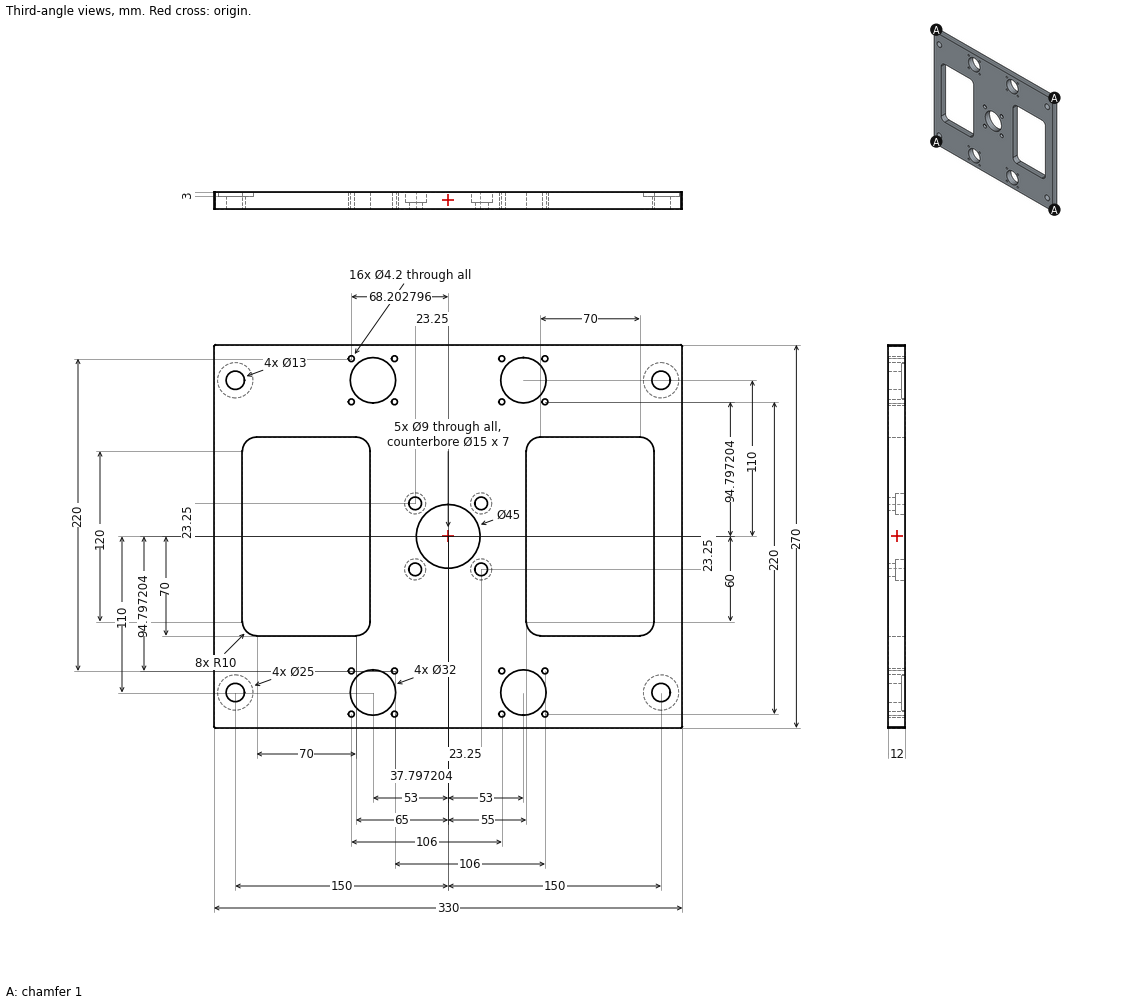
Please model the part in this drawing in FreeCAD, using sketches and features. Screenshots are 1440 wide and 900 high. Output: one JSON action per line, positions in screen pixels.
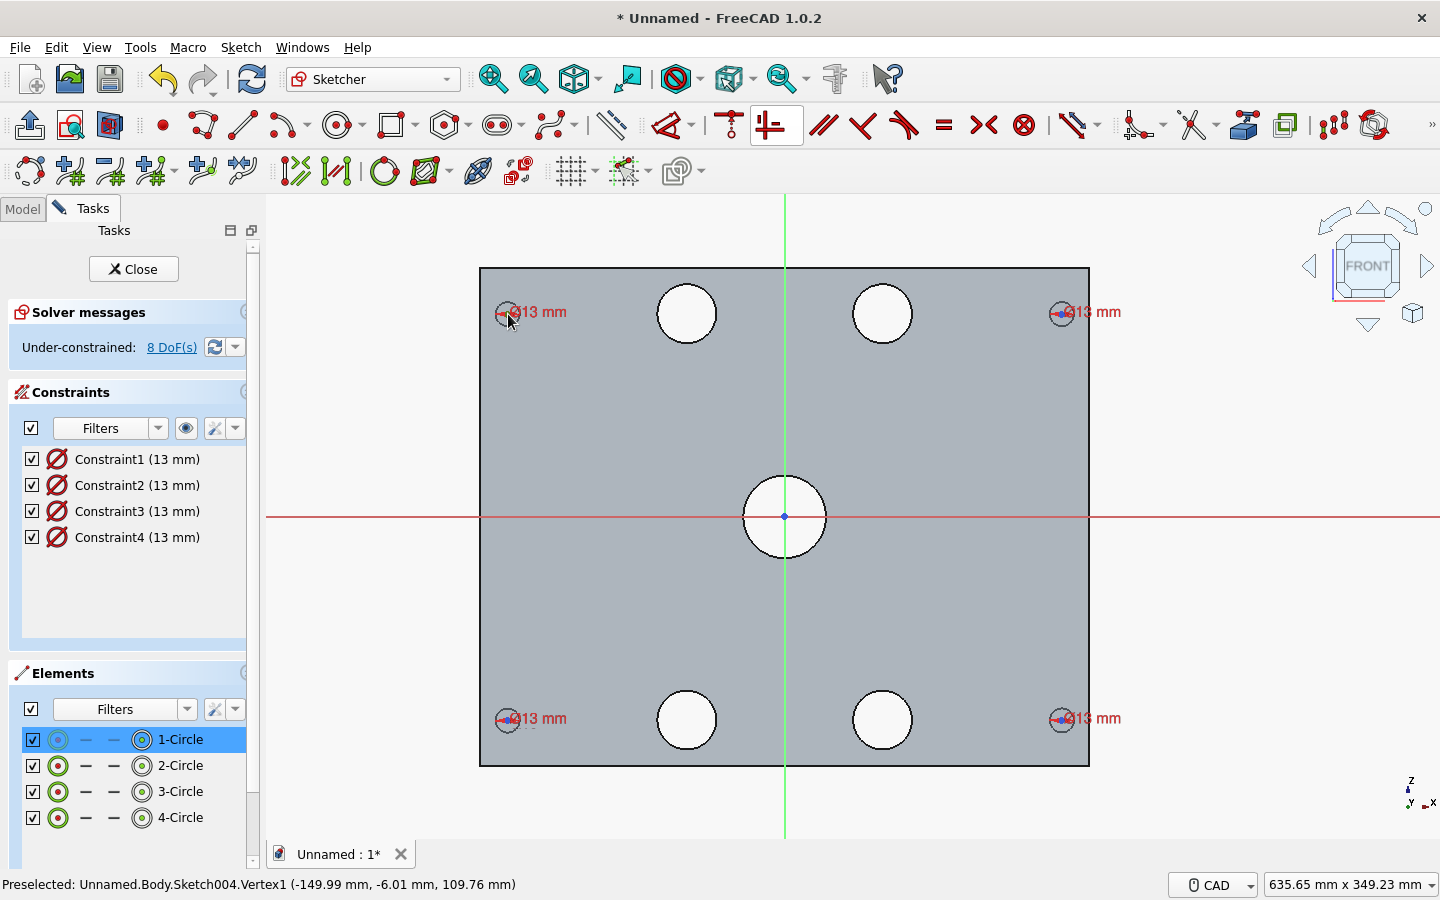
{"action": "left_click", "coordinate": [1062, 314]}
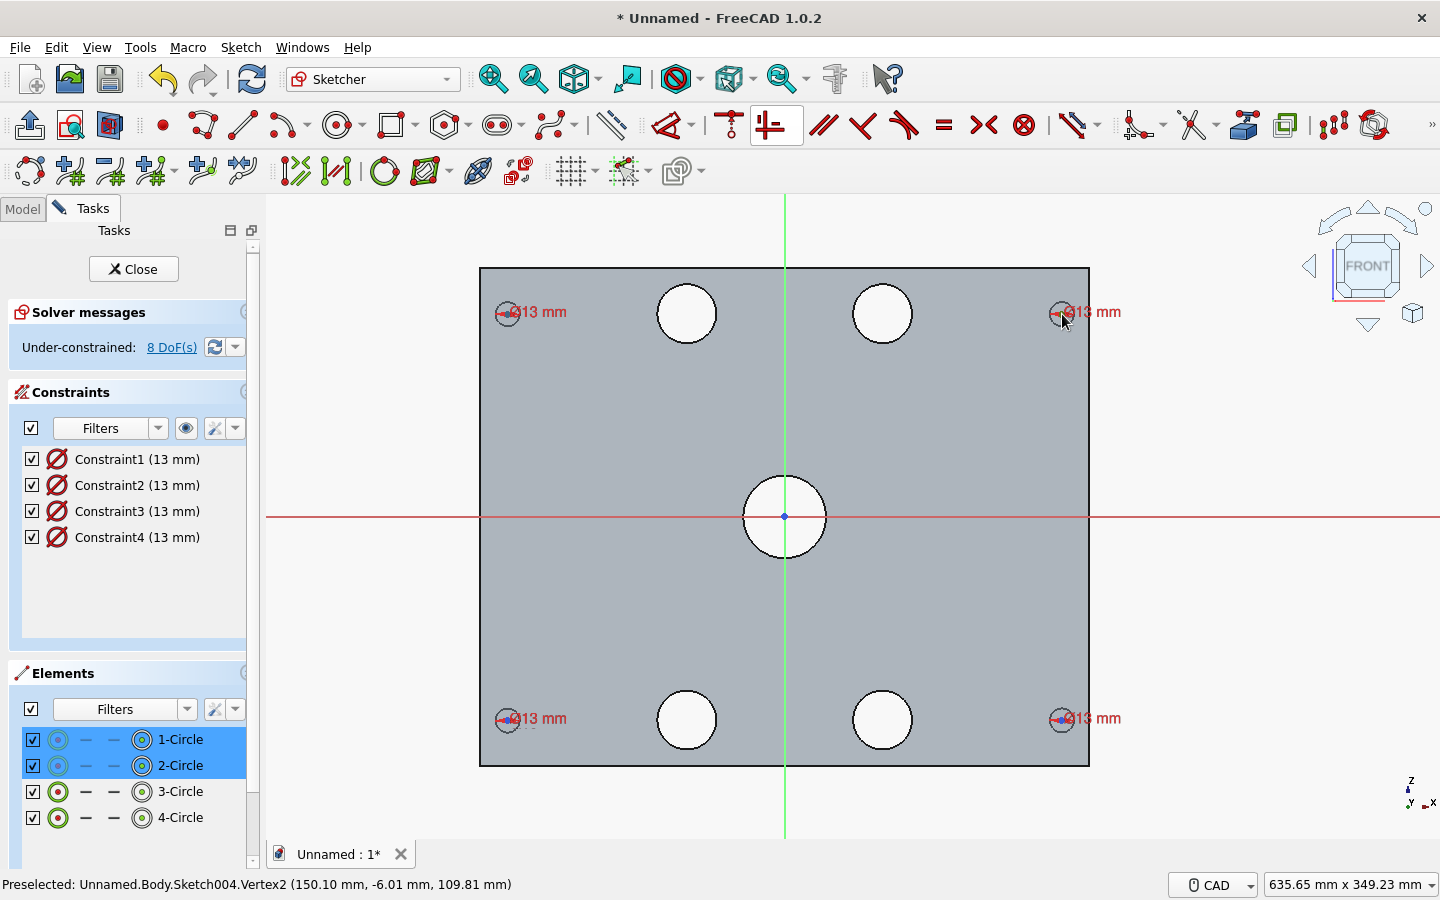
{"action": "key", "text": "h"}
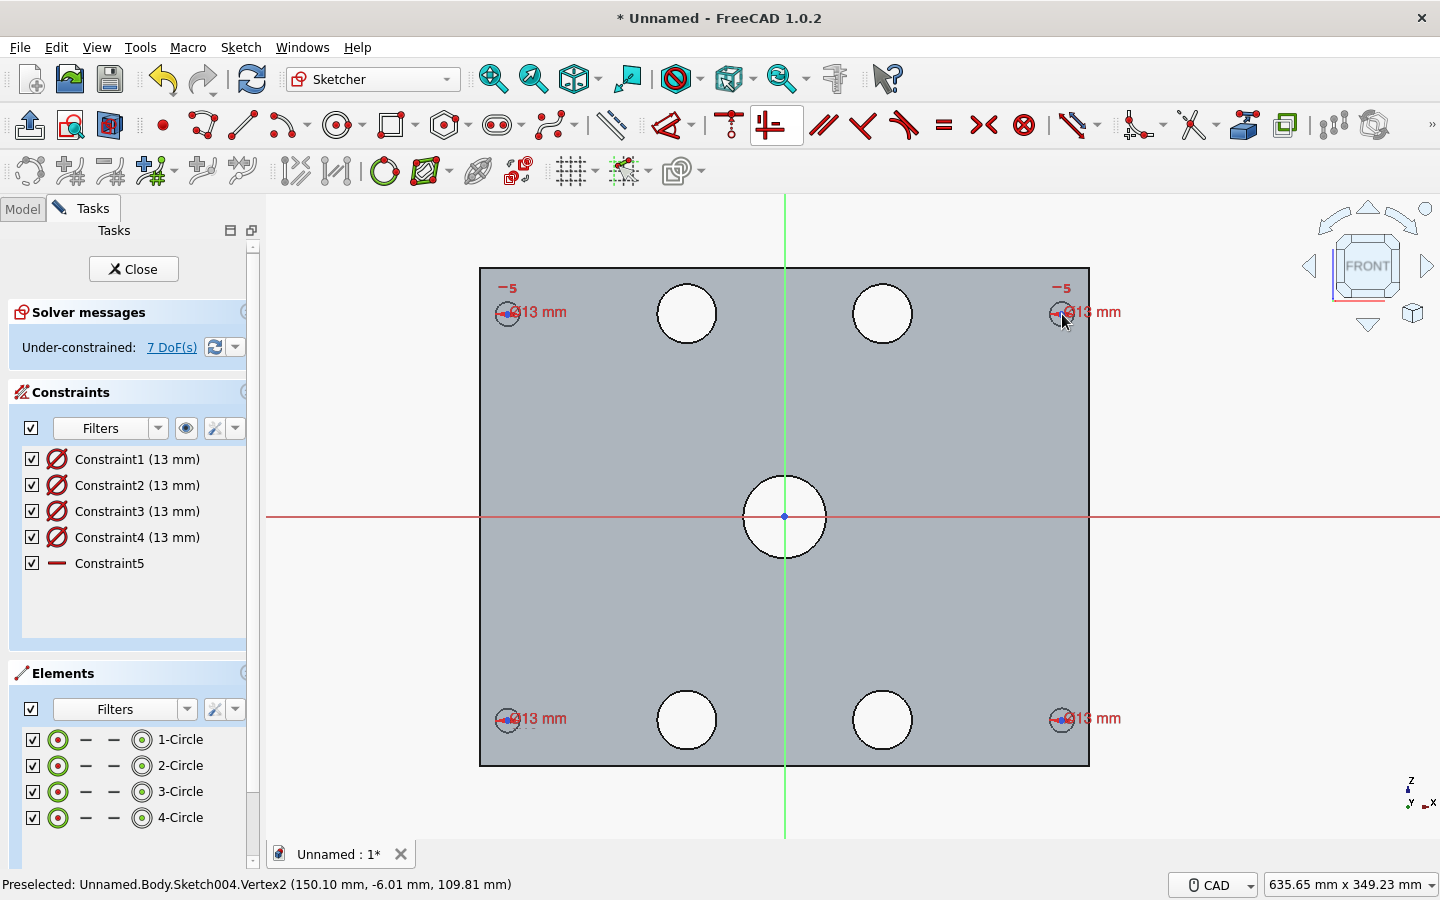
{"action": "left_click", "coordinate": [508, 314]}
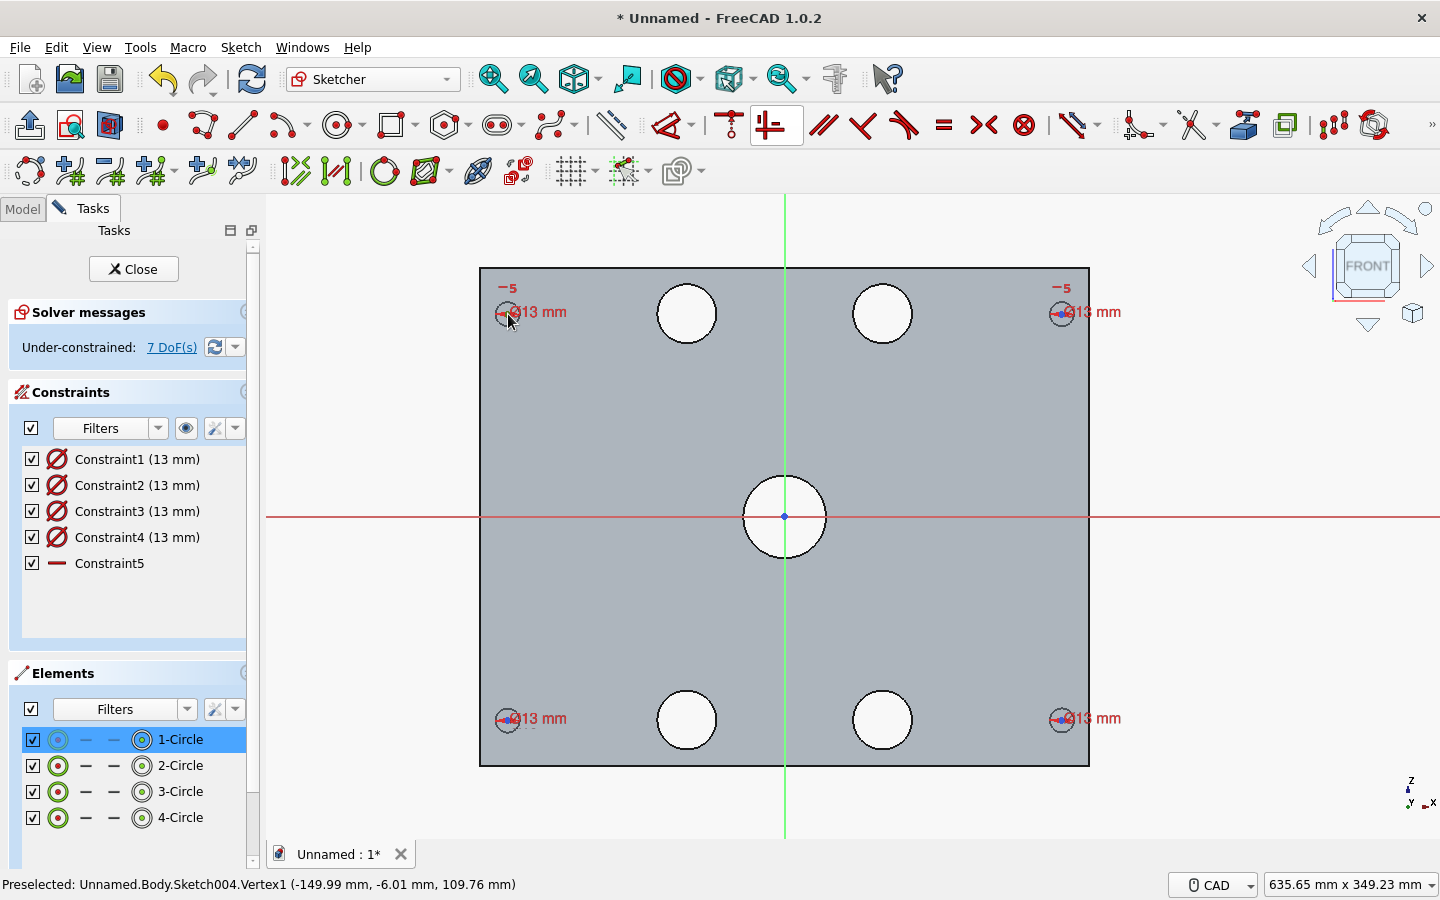
{"action": "left_click", "coordinate": [508, 721]}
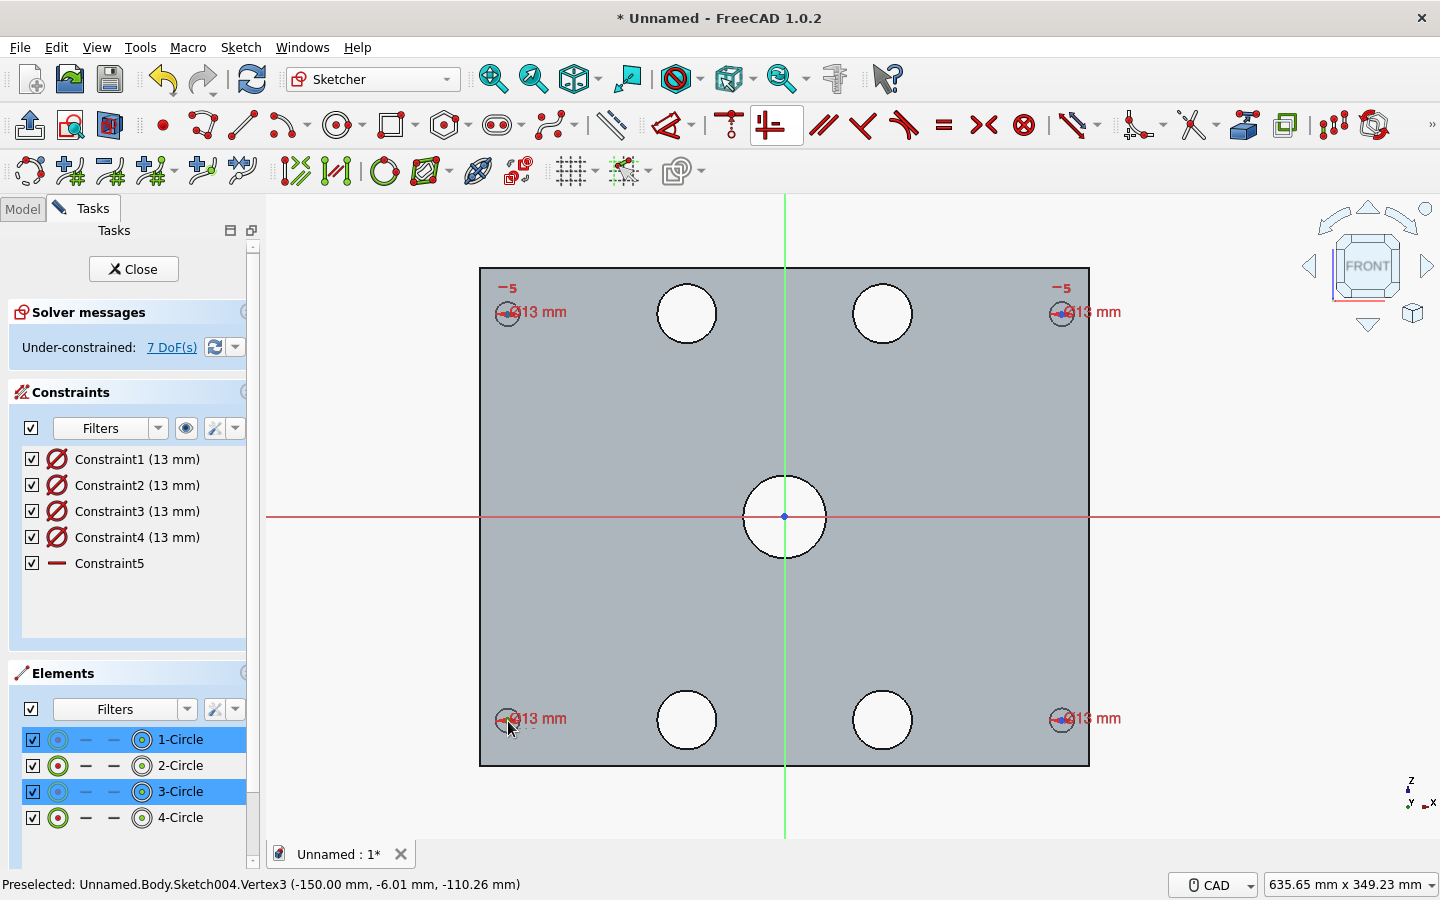
{"action": "left_click", "coordinate": [798, 126]}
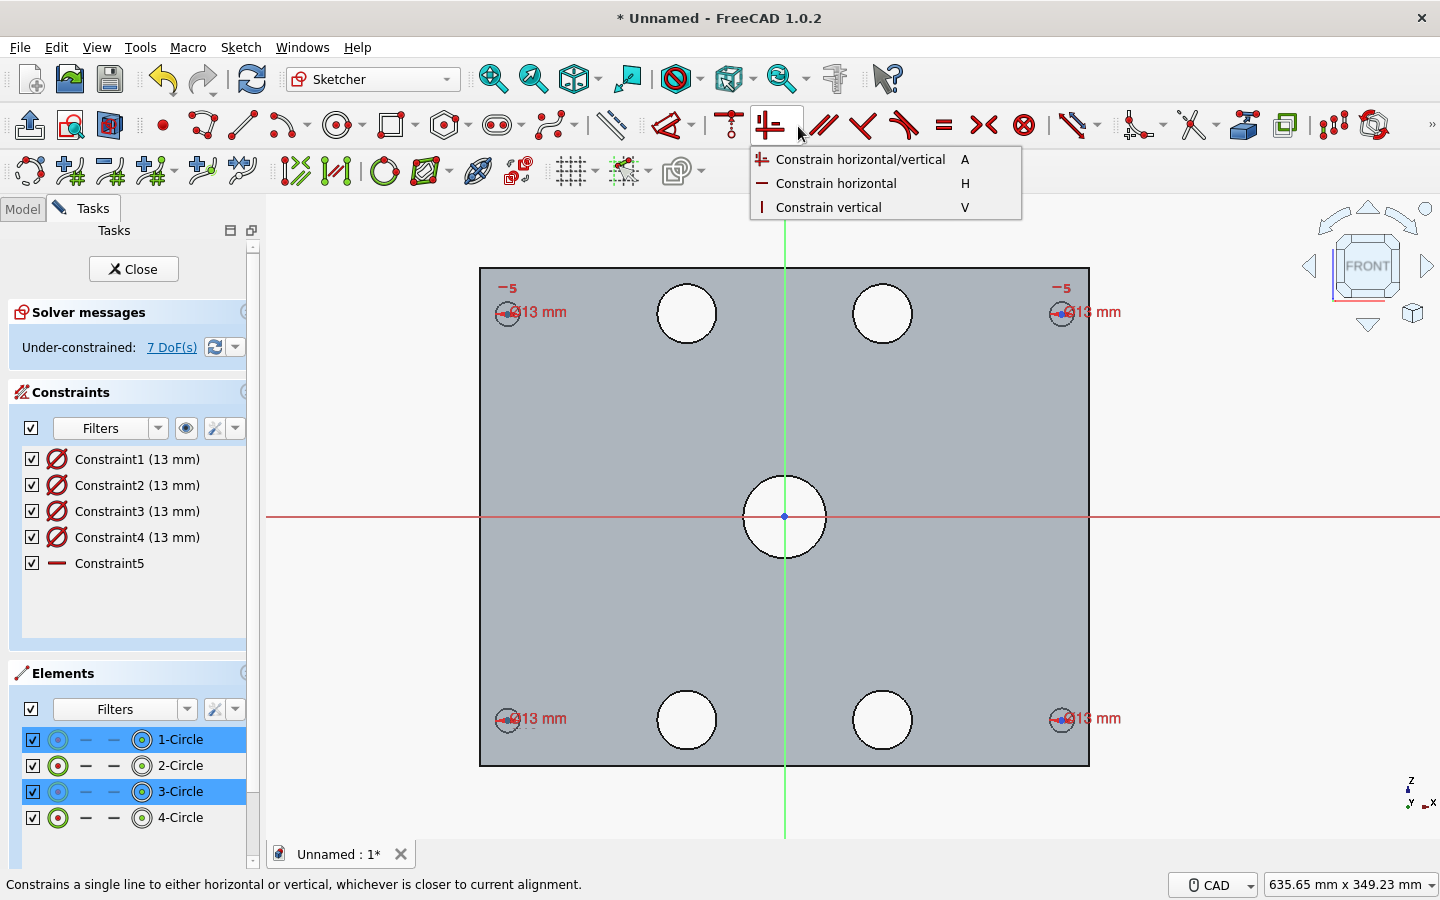
{"action": "left_click", "coordinate": [886, 207]}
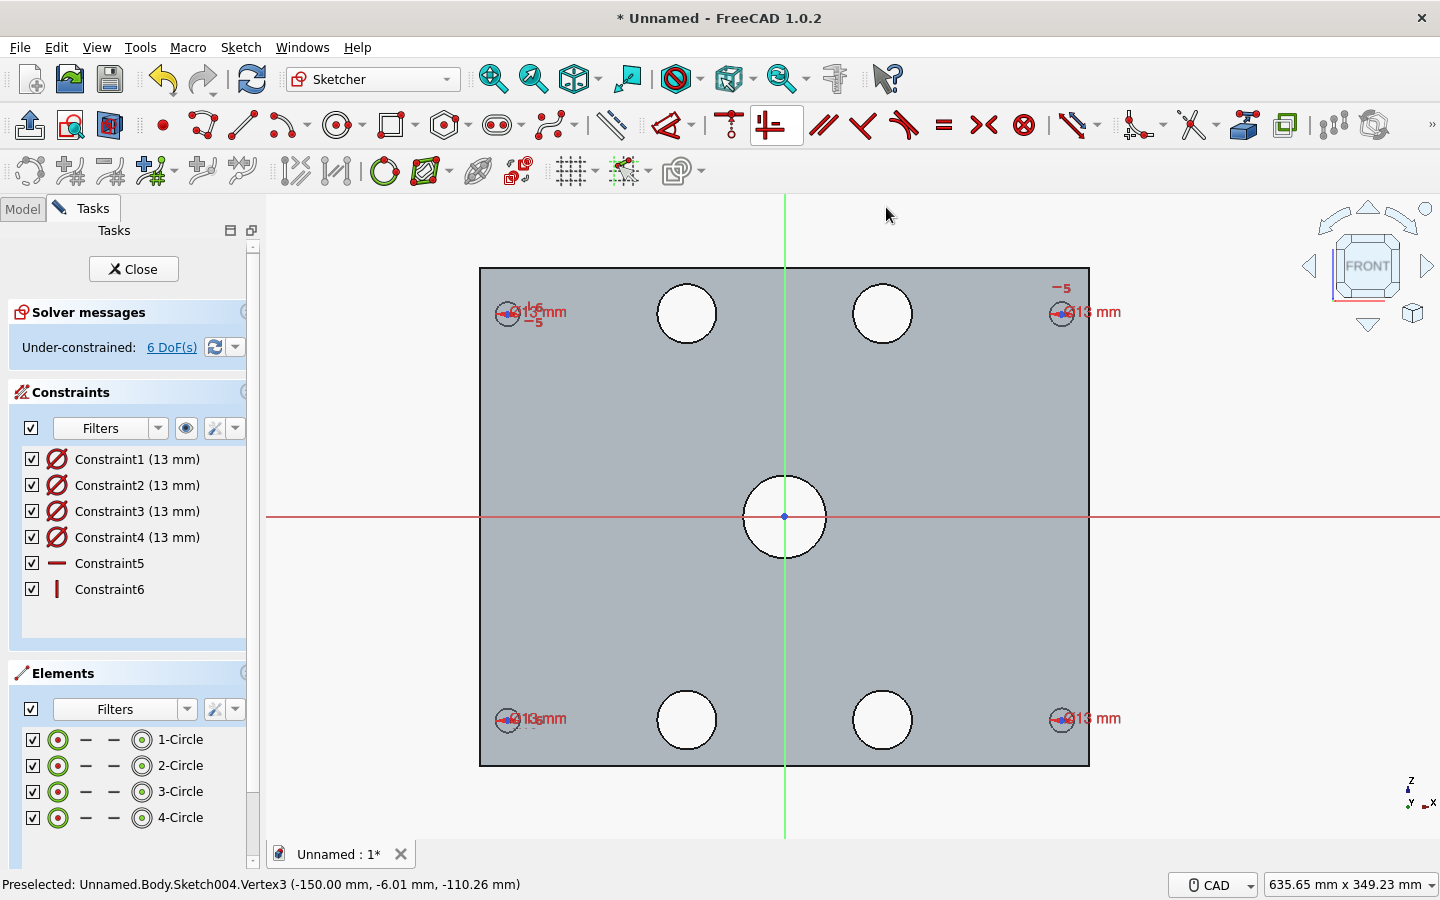
{"action": "left_click", "coordinate": [1062, 314]}